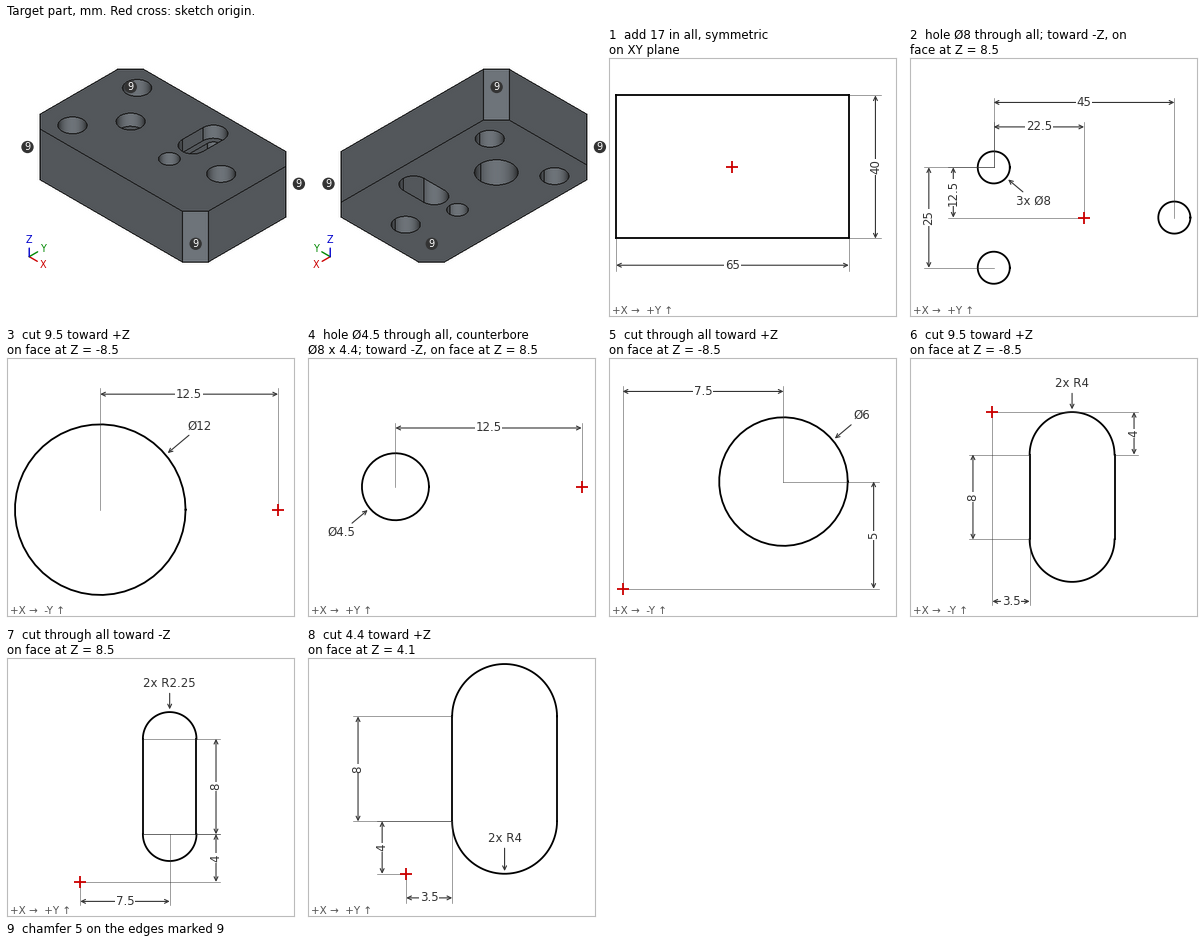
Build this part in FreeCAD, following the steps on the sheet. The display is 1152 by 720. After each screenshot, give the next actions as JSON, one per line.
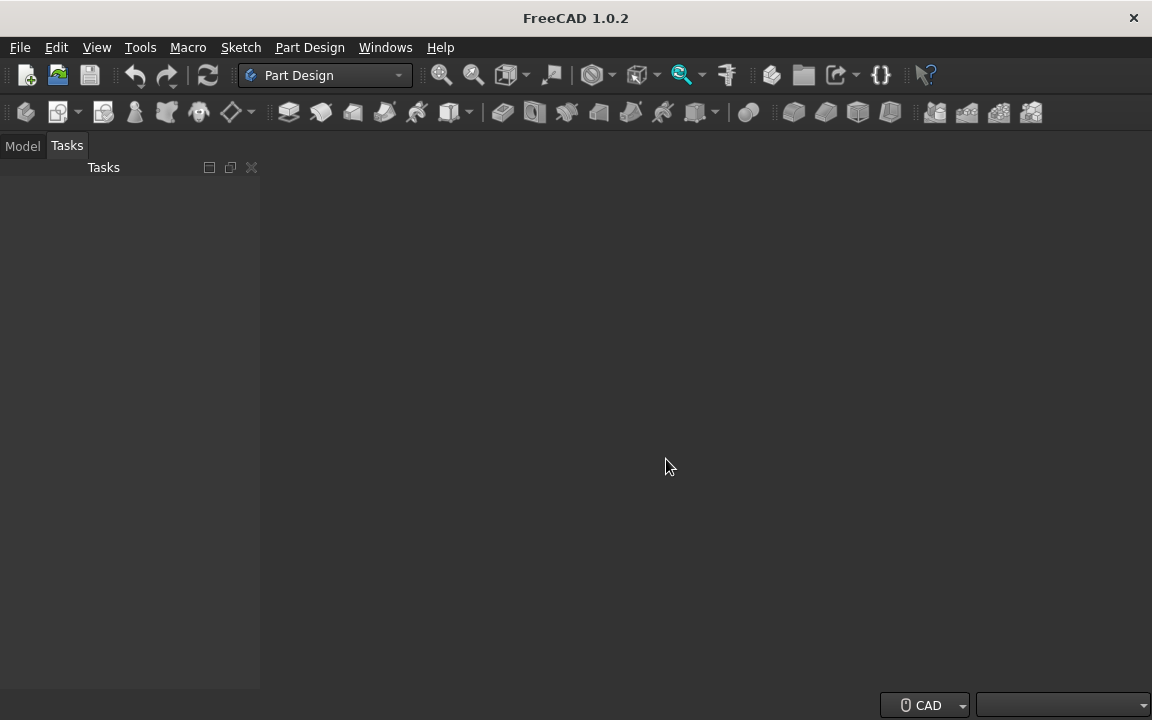
{"action": "left_click", "coordinate": [26, 76]}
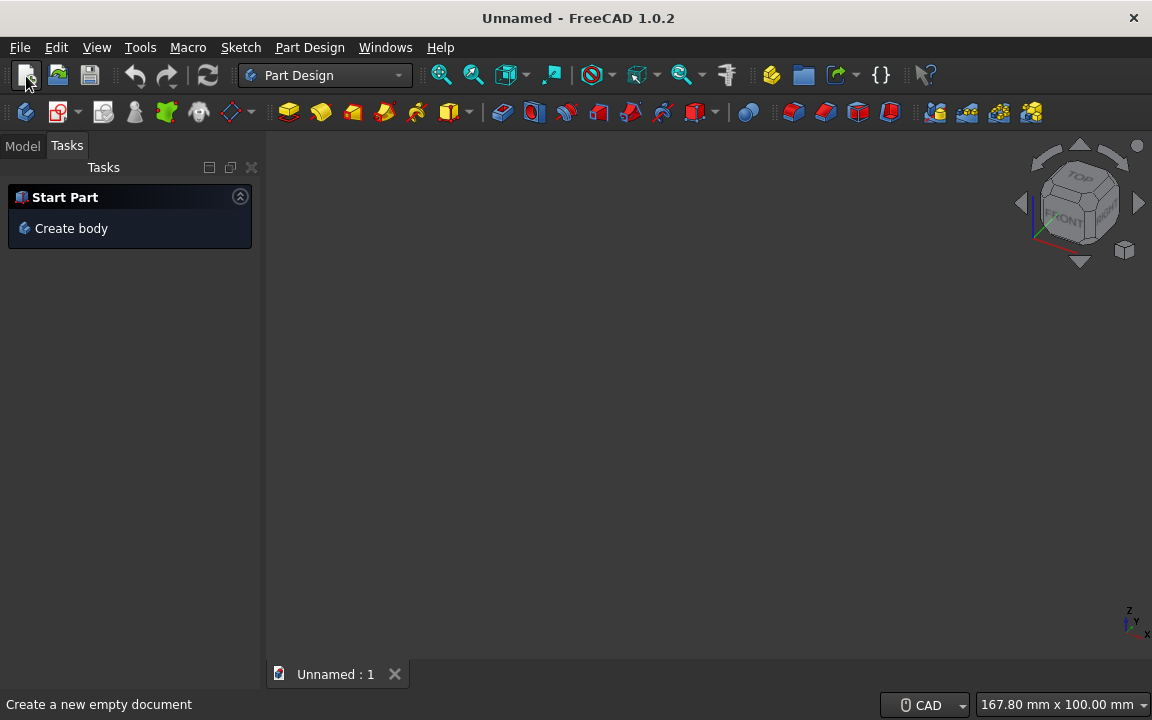
{"action": "left_click", "coordinate": [58, 112]}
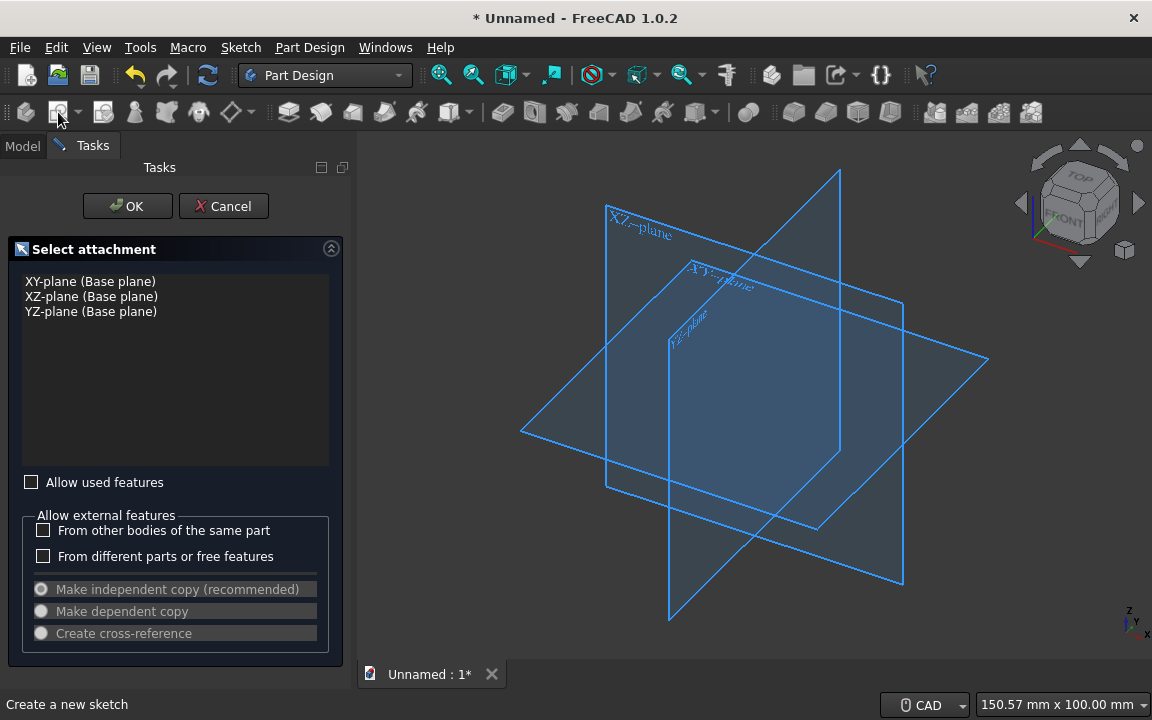
{"action": "left_click", "coordinate": [82, 282]}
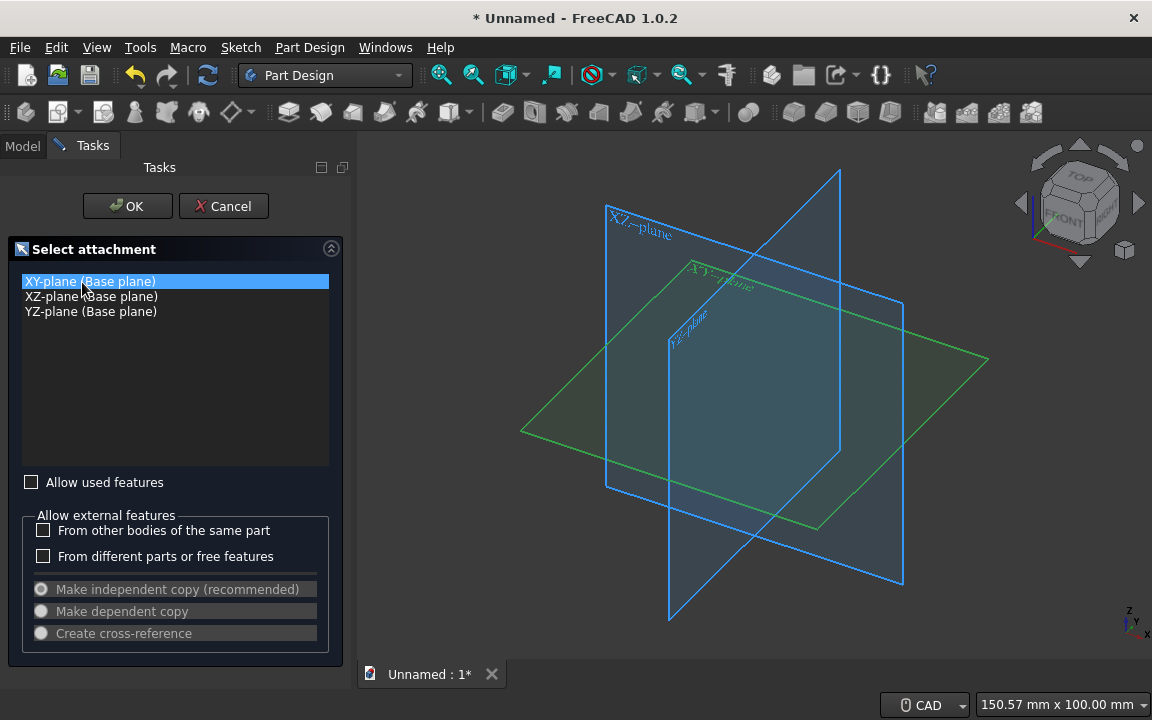
{"action": "left_click", "coordinate": [128, 206]}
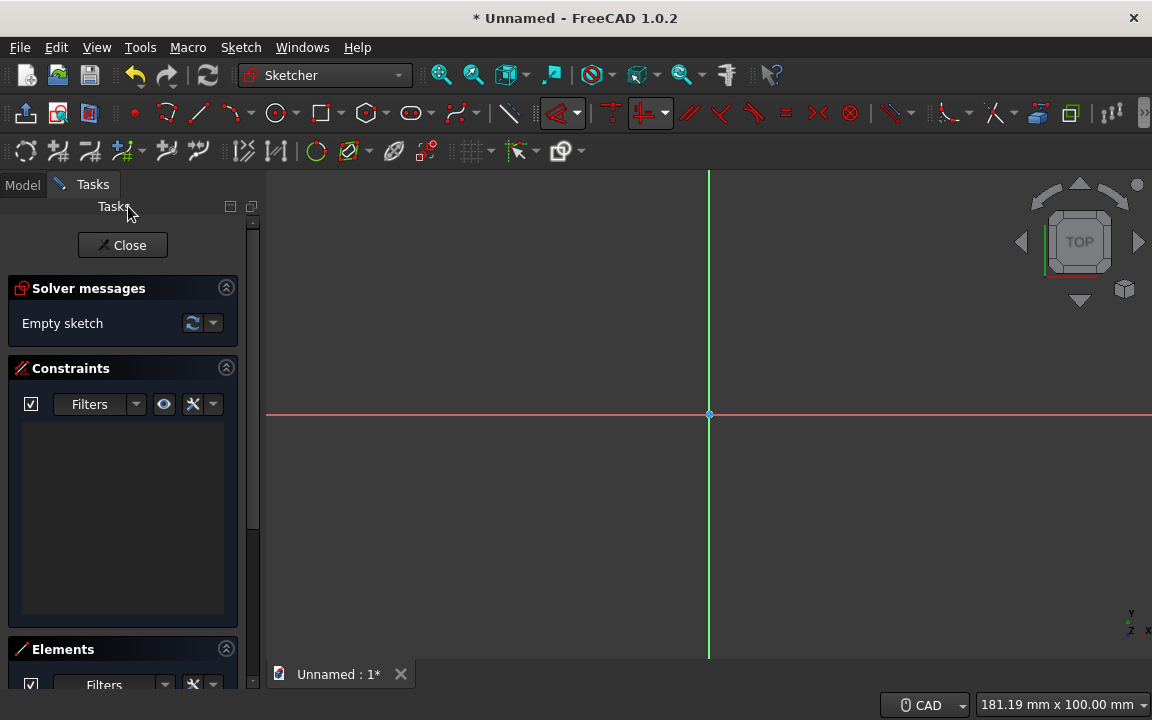
{"action": "scroll", "coordinate": [848, 414], "scroll_direction": "up", "scroll_amount": 2}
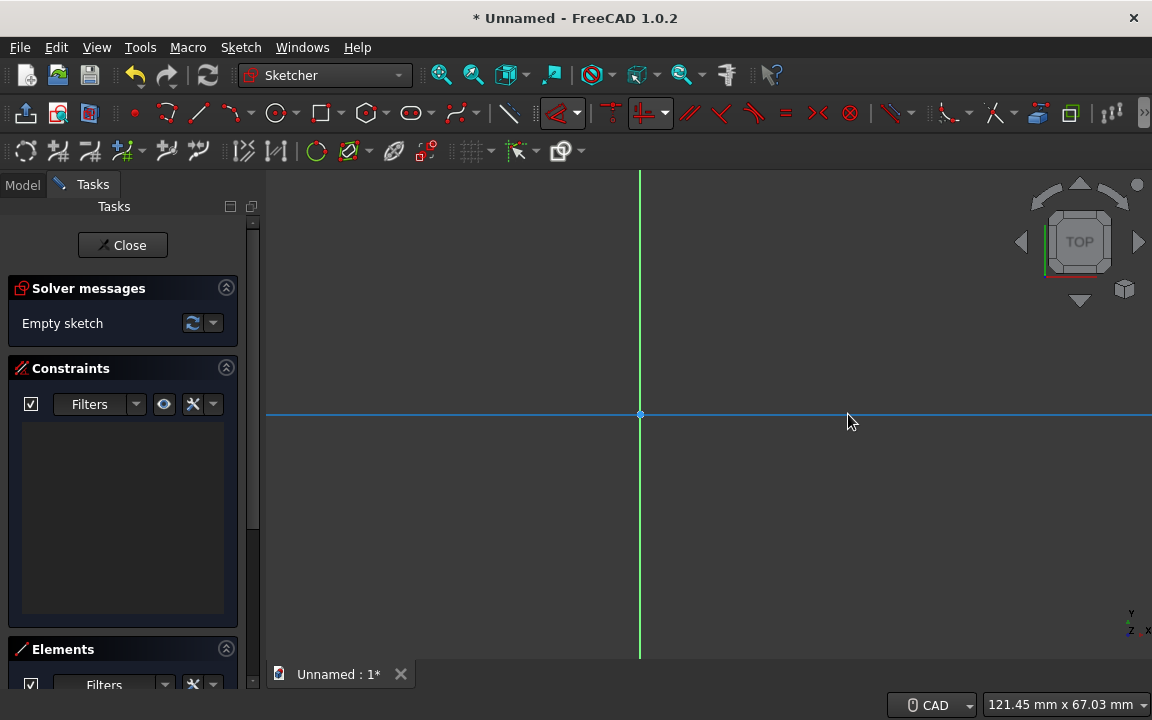
{"action": "key", "text": "g v"}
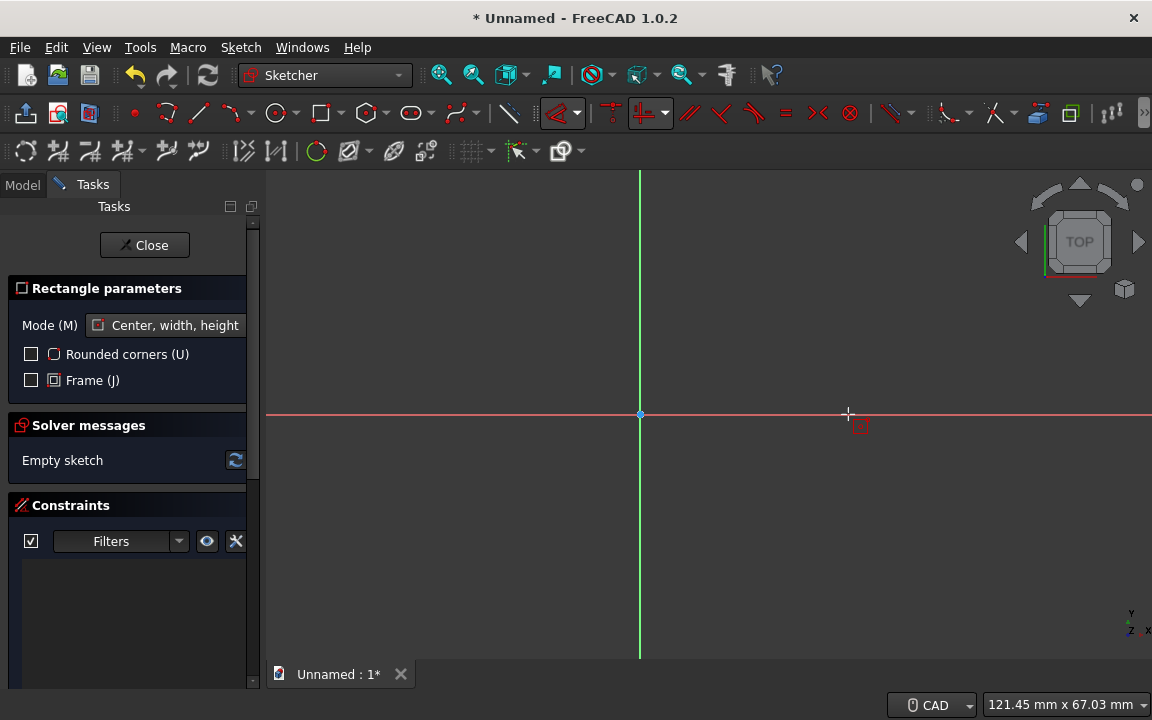
{"action": "left_click", "coordinate": [640, 414]}
{"action": "left_click", "coordinate": [877, 269]}
{"action": "key", "text": "Escape"}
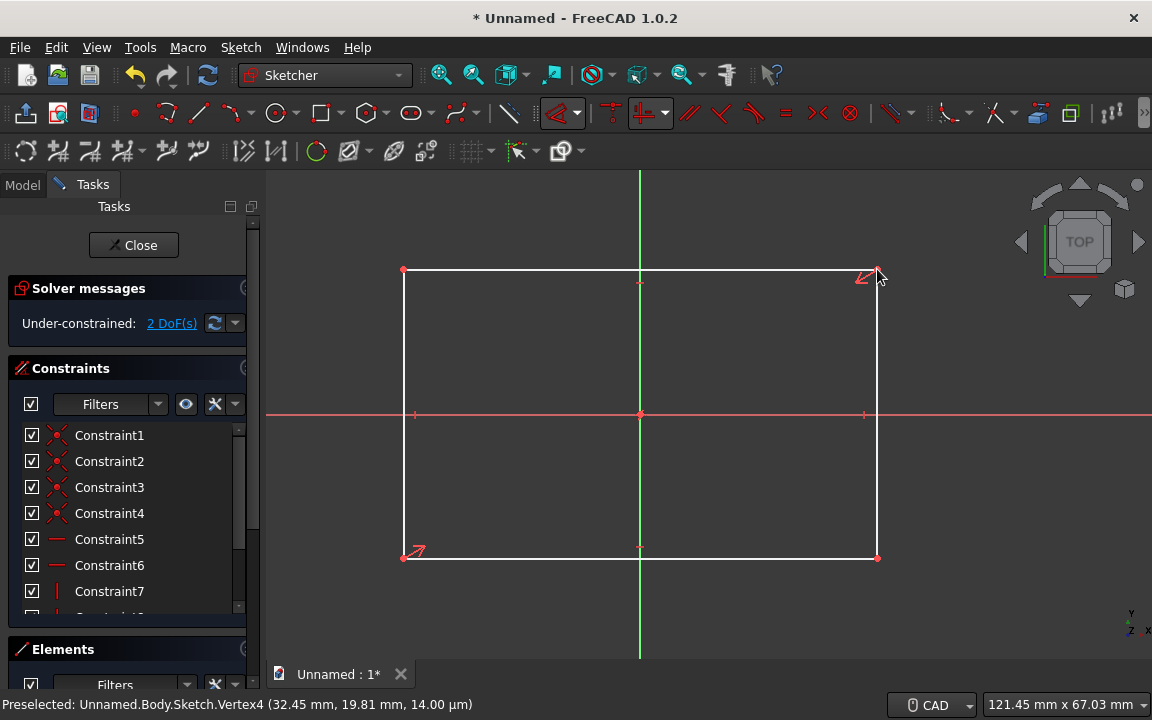
{"action": "key", "text": "d"}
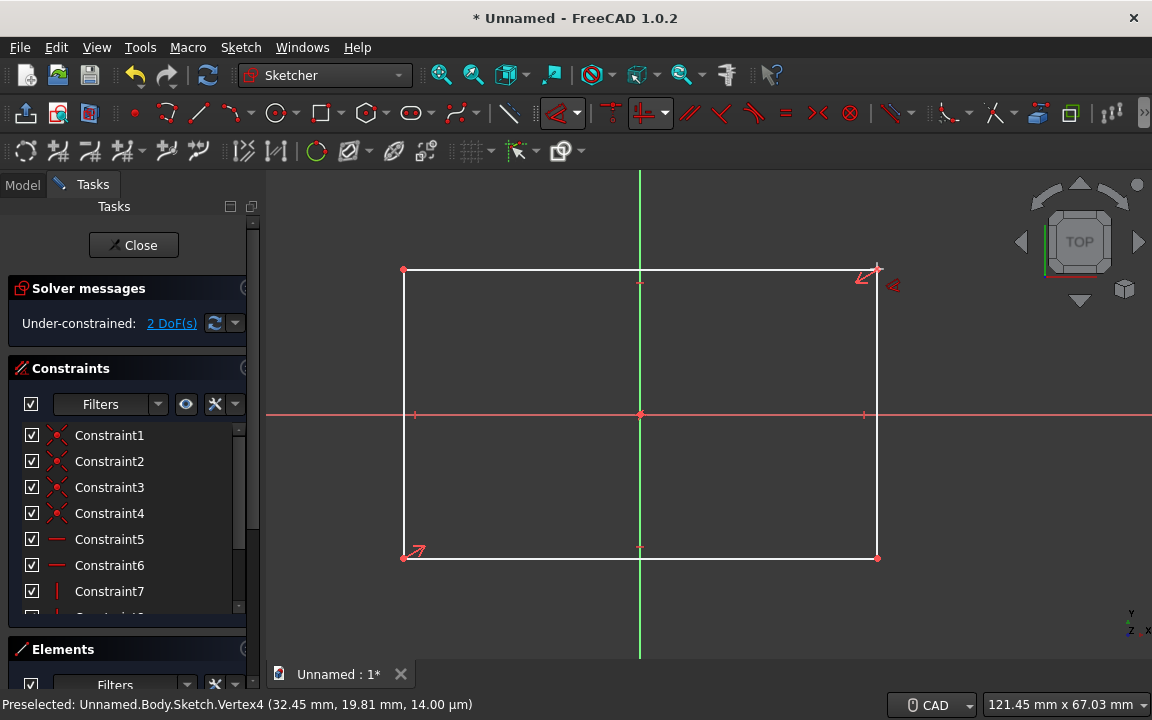
{"action": "left_click", "coordinate": [546, 559]}
{"action": "left_click", "coordinate": [531, 593]}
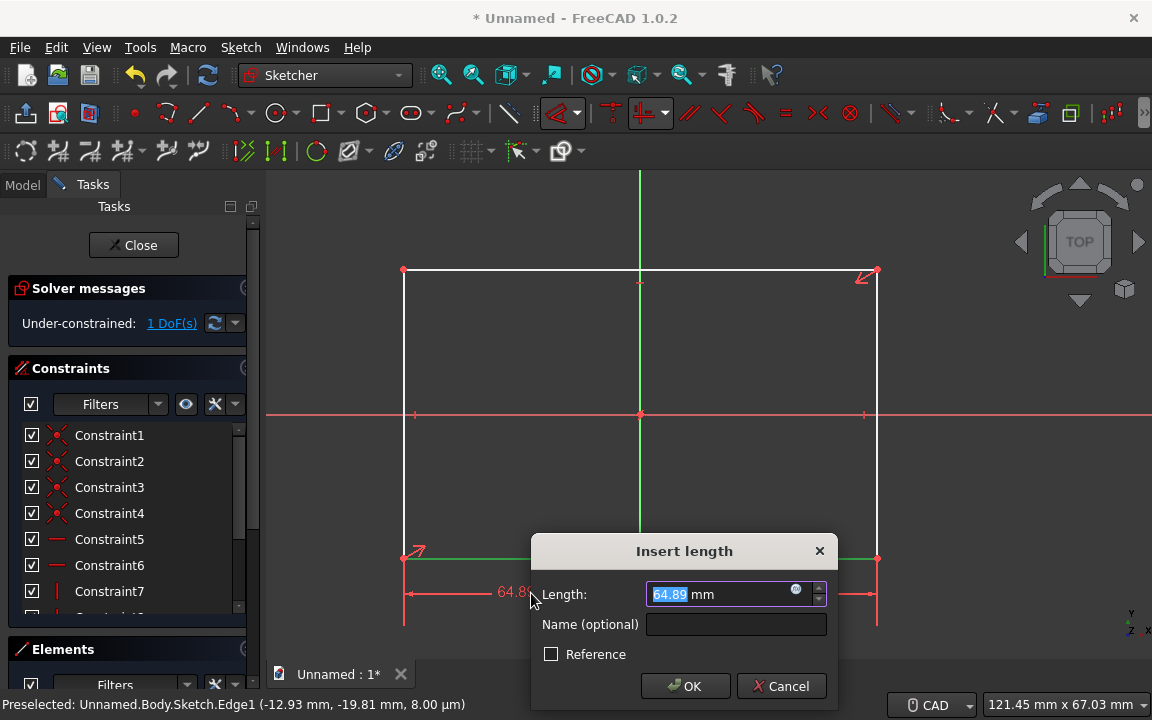
{"action": "type", "text": "65"}
{"action": "key", "text": "Return"}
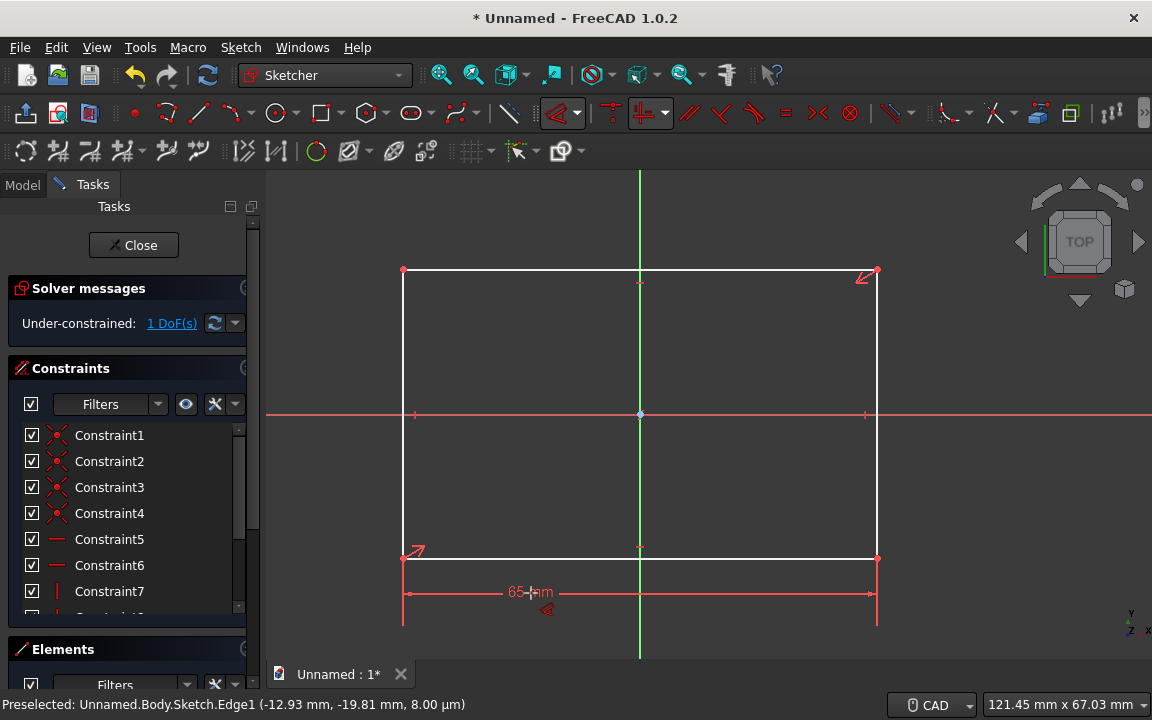
{"action": "left_click", "coordinate": [877, 472]}
{"action": "left_click", "coordinate": [911, 348]}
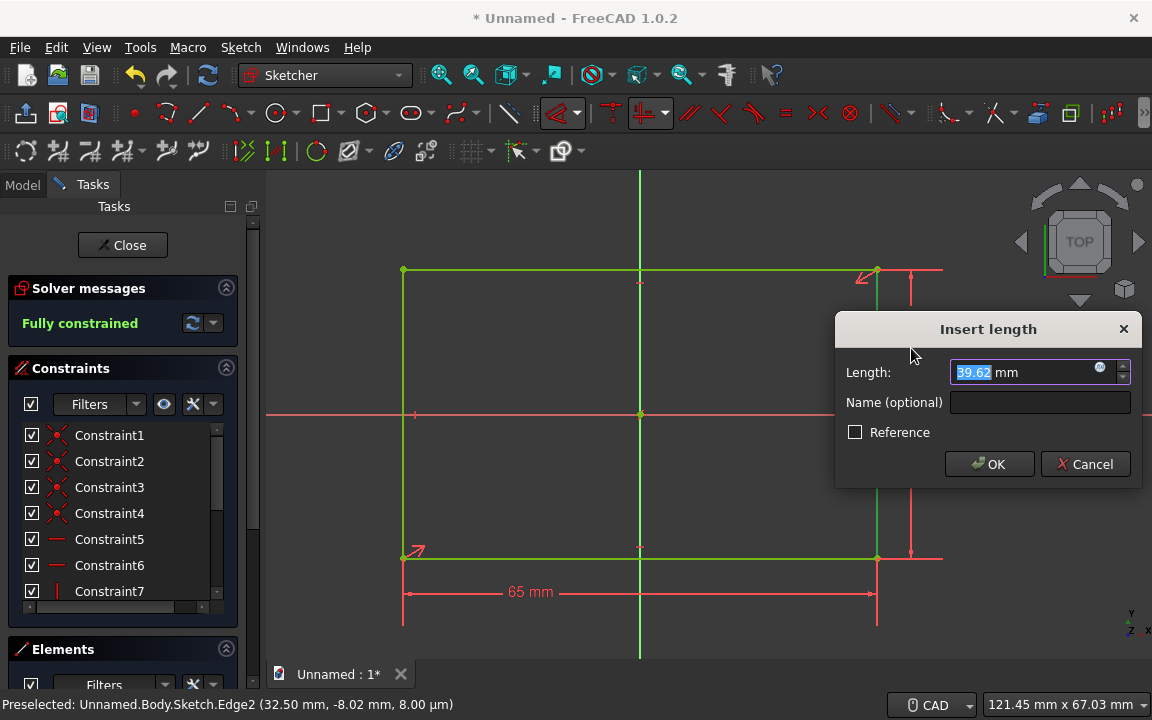
{"action": "type", "text": "40"}
{"action": "key", "text": "Return"}
{"action": "key", "text": "Escape"}